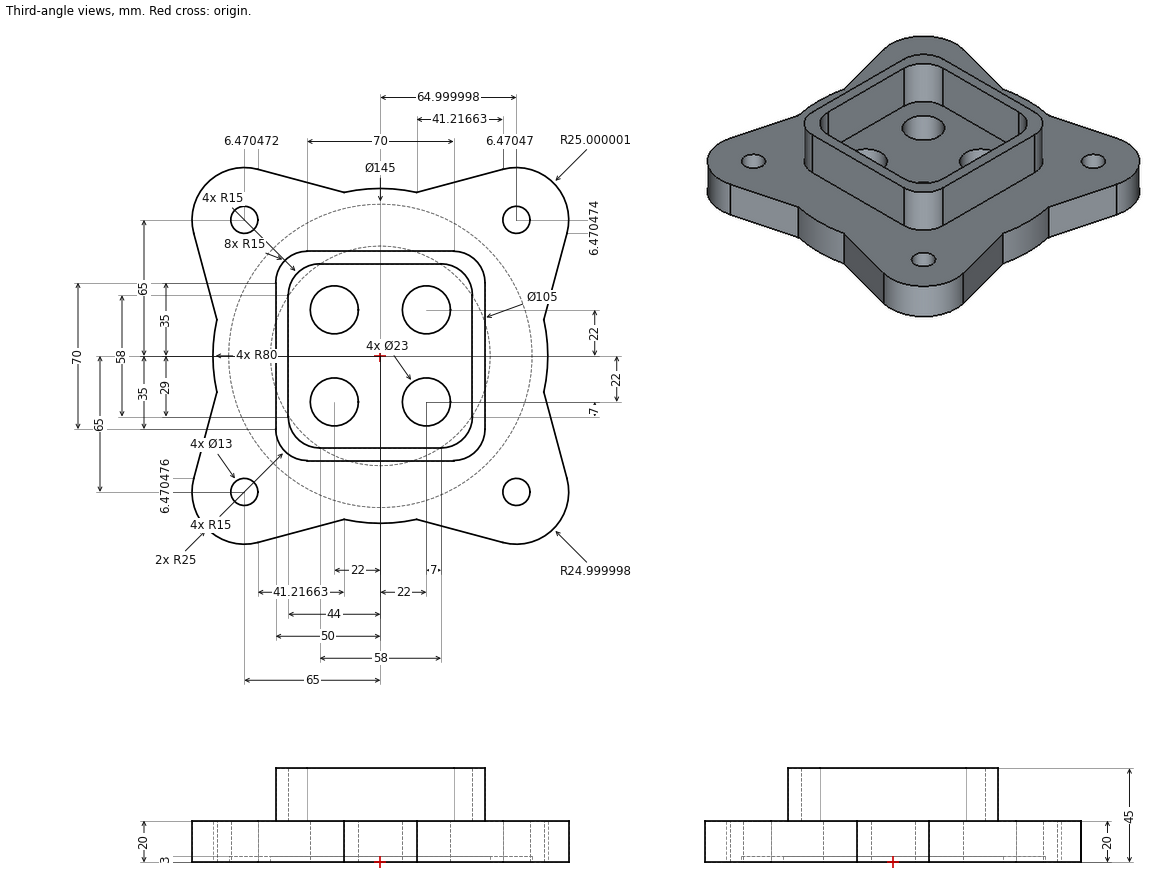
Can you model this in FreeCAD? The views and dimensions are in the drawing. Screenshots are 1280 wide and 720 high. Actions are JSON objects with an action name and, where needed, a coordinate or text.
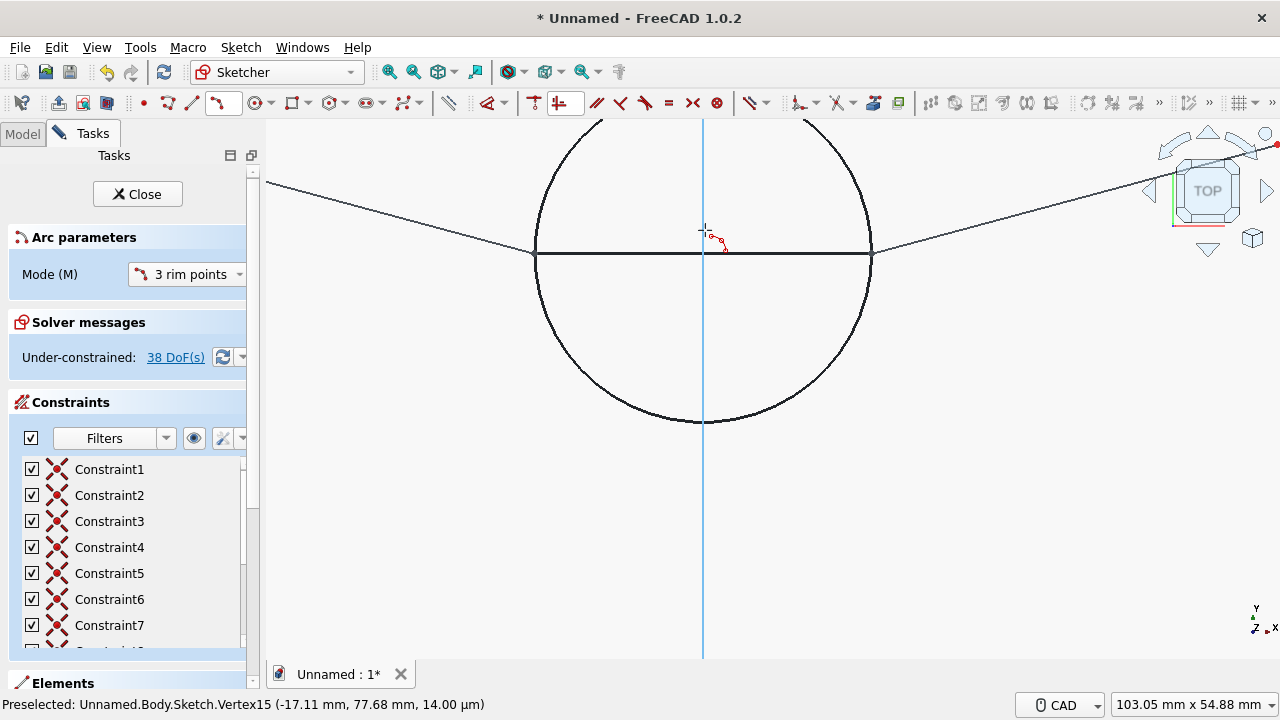
{"action": "left_click", "coordinate": [703, 231]}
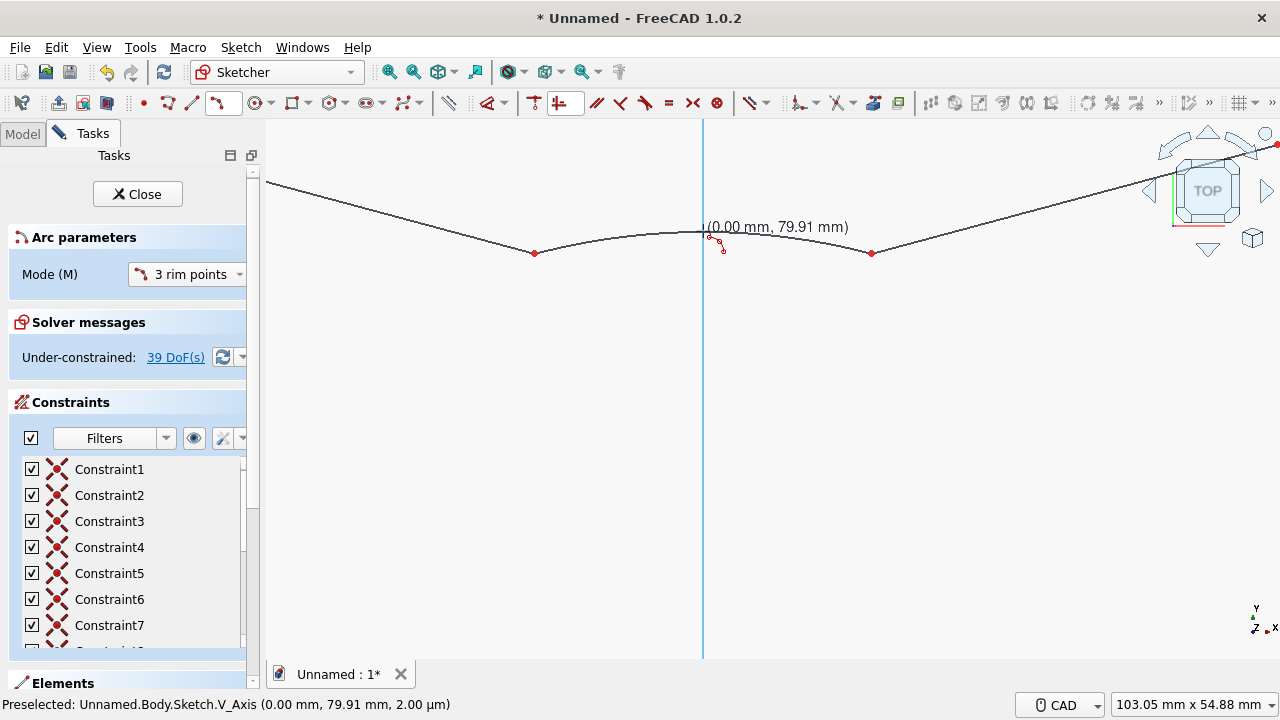
{"action": "scroll", "coordinate": [705, 230], "scroll_direction": "down", "scroll_amount": 8}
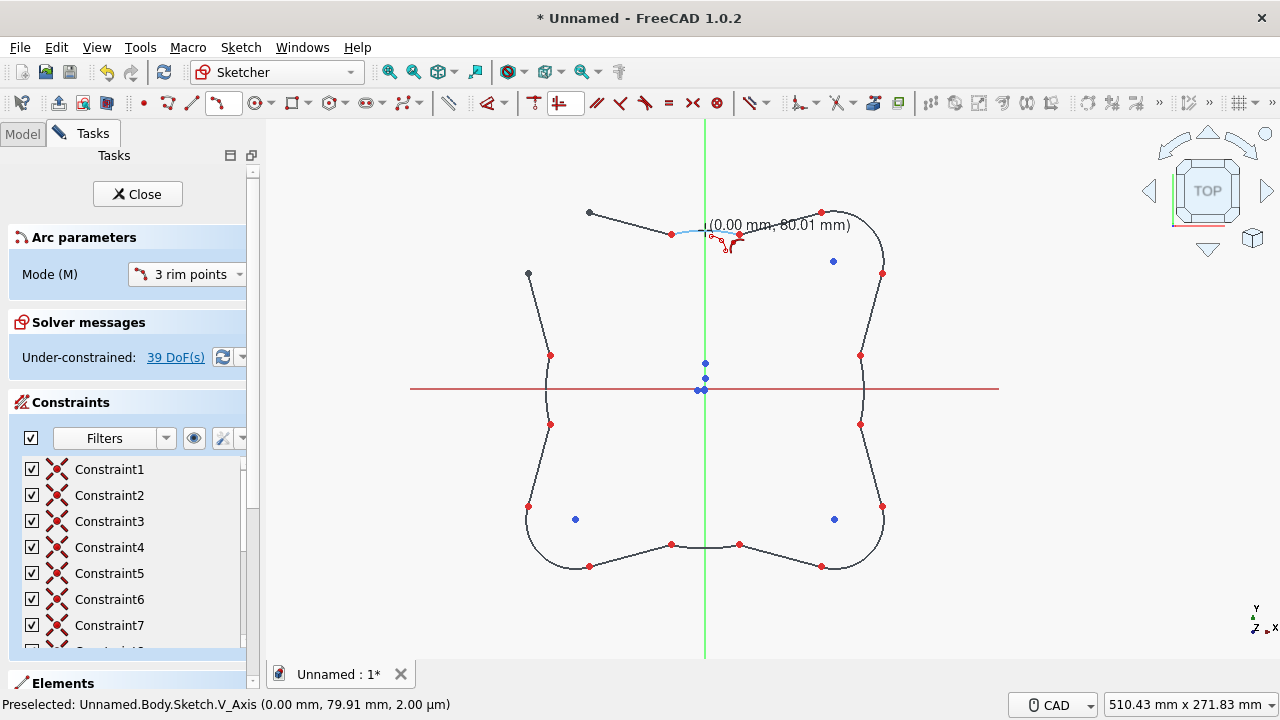
{"action": "left_click", "coordinate": [589, 213]}
{"action": "left_click", "coordinate": [528, 274]}
{"action": "left_click", "coordinate": [541, 225]}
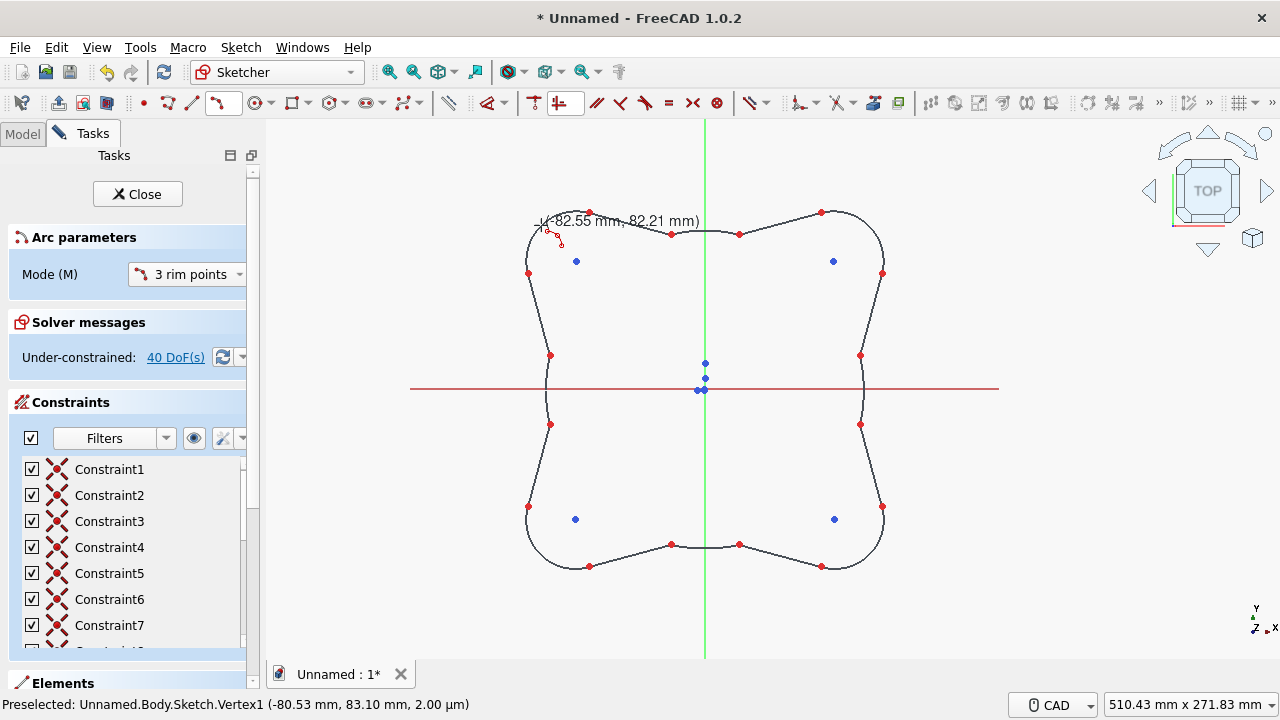
{"action": "left_click", "coordinate": [192, 104]}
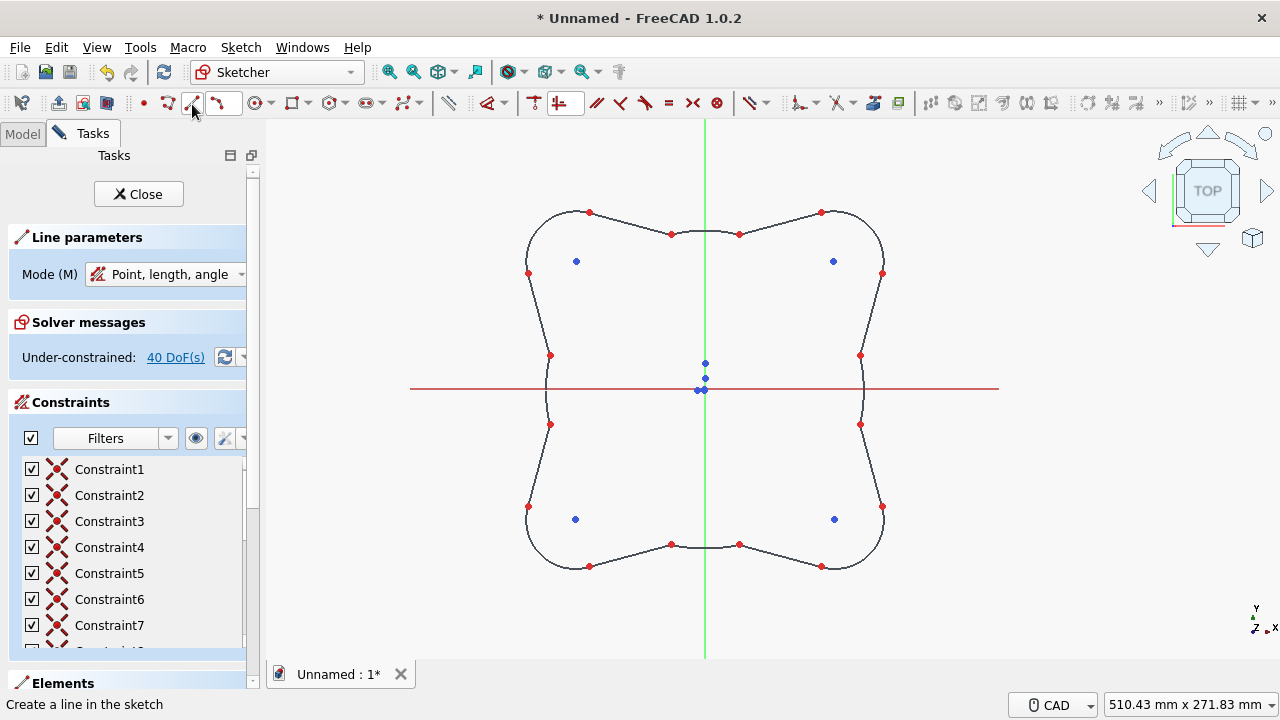
{"action": "left_click", "coordinate": [606, 459]}
{"action": "left_click", "coordinate": [606, 320]}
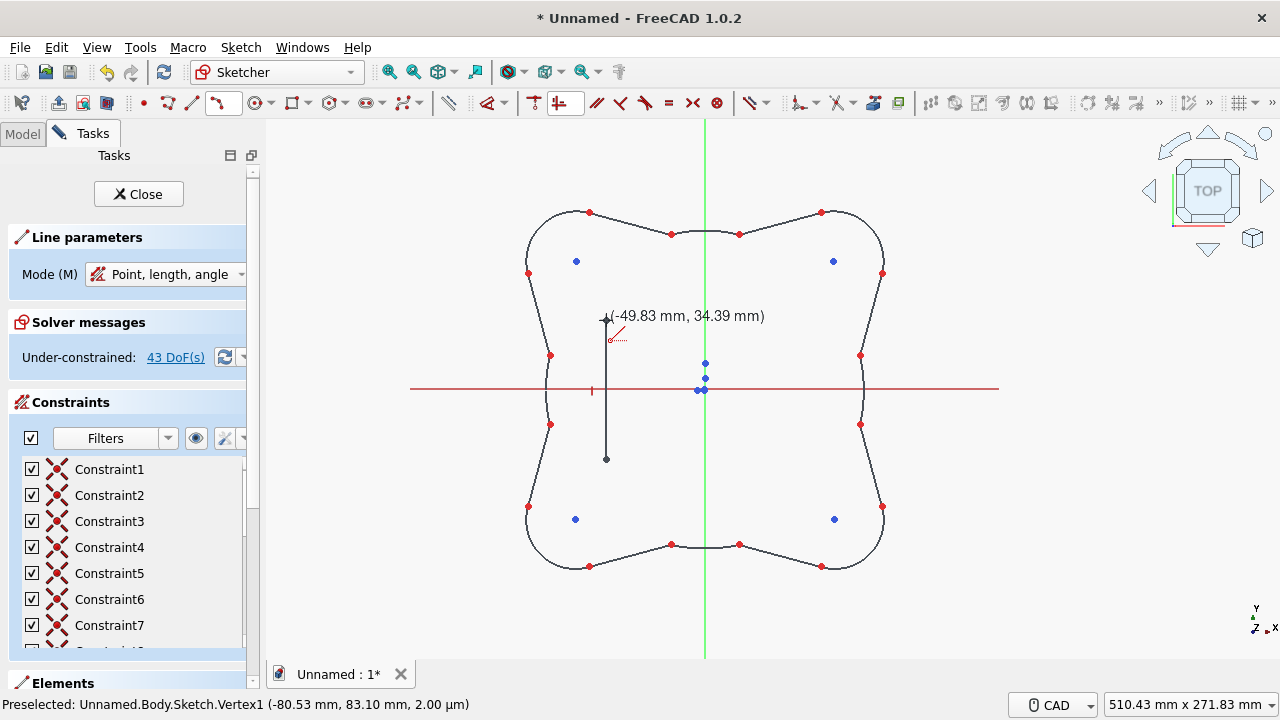
{"action": "left_click", "coordinate": [635, 290]}
{"action": "left_click", "coordinate": [775, 290]}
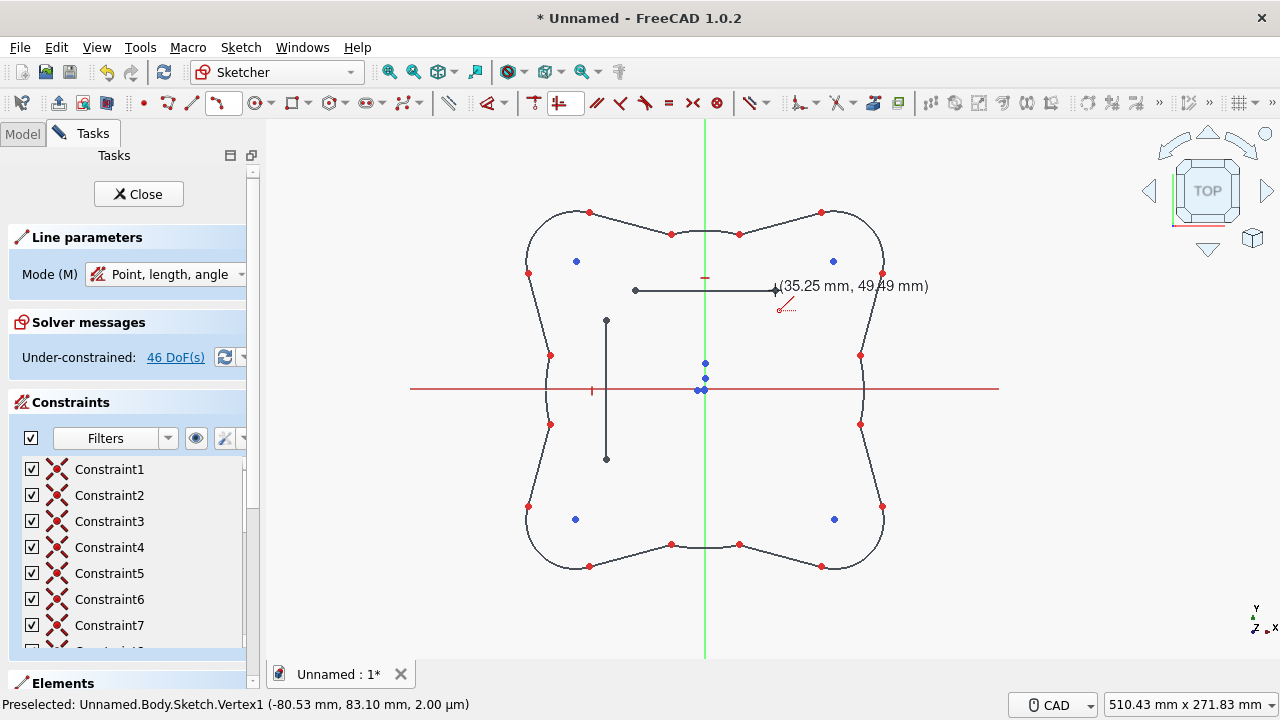
{"action": "left_click", "coordinate": [804, 320]}
{"action": "left_click", "coordinate": [804, 459]}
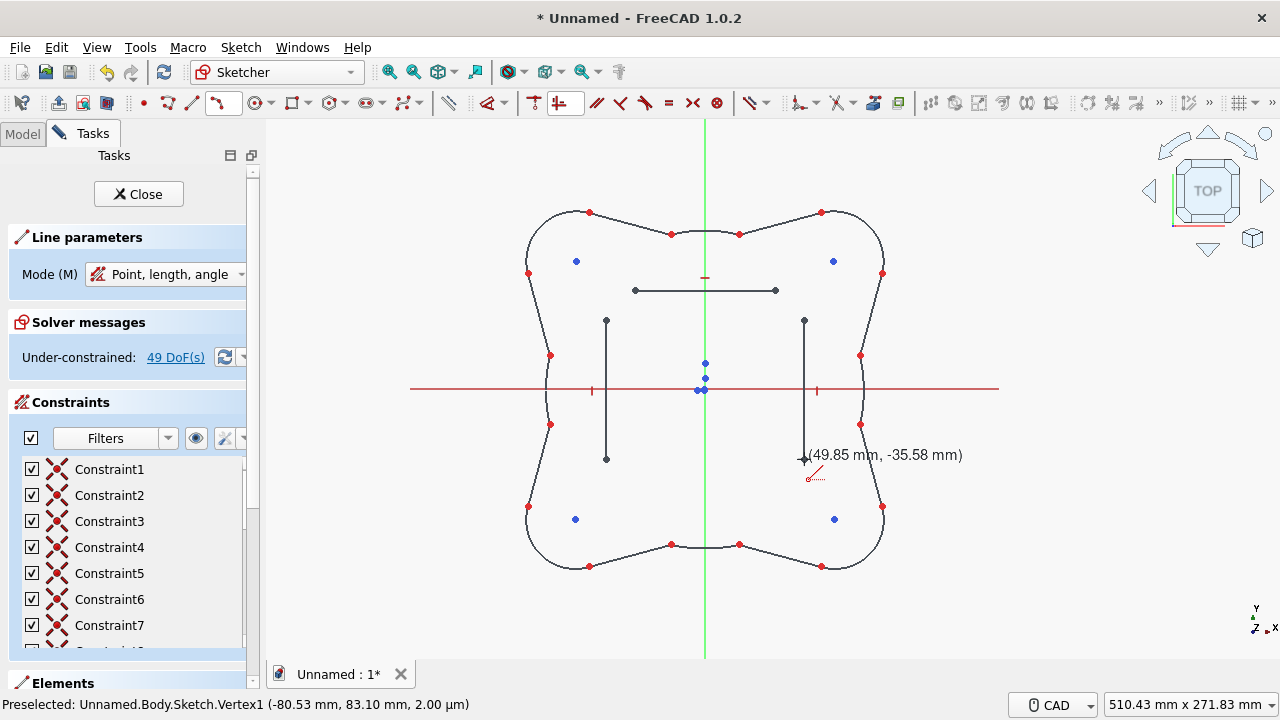
{"action": "left_click", "coordinate": [775, 489]}
{"action": "left_click", "coordinate": [635, 489]}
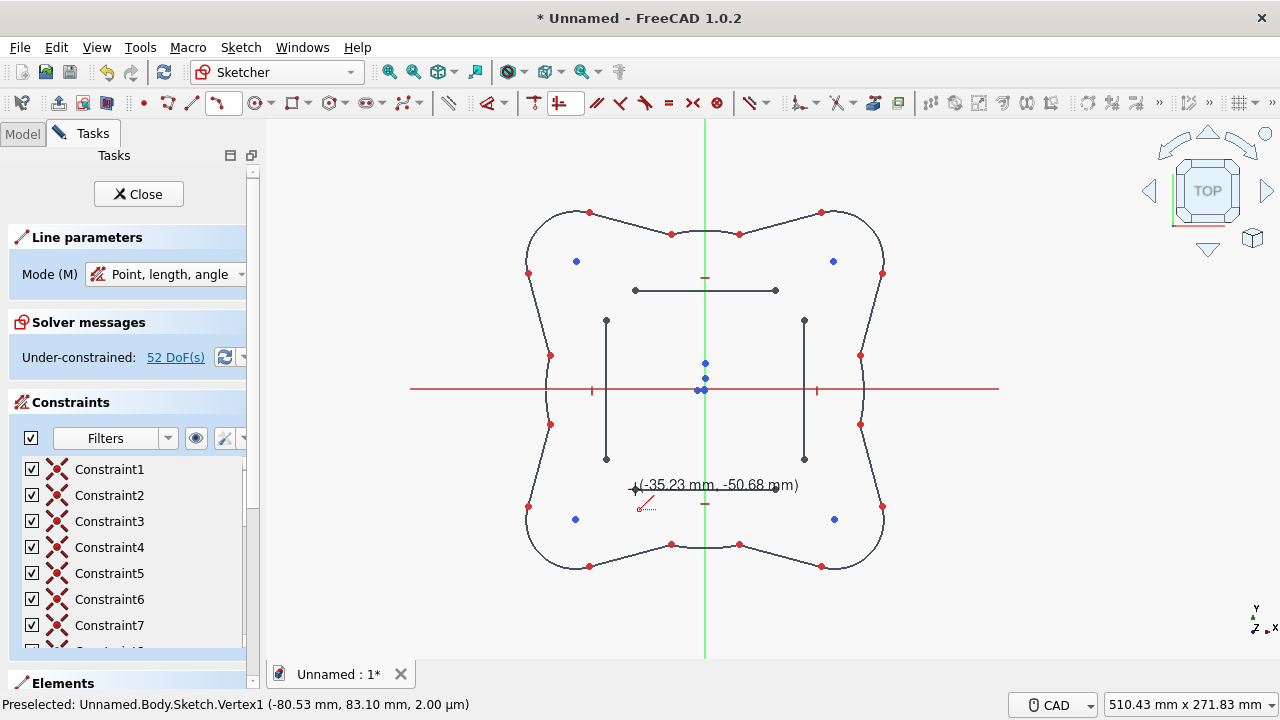
{"action": "key", "text": "g 3 a"}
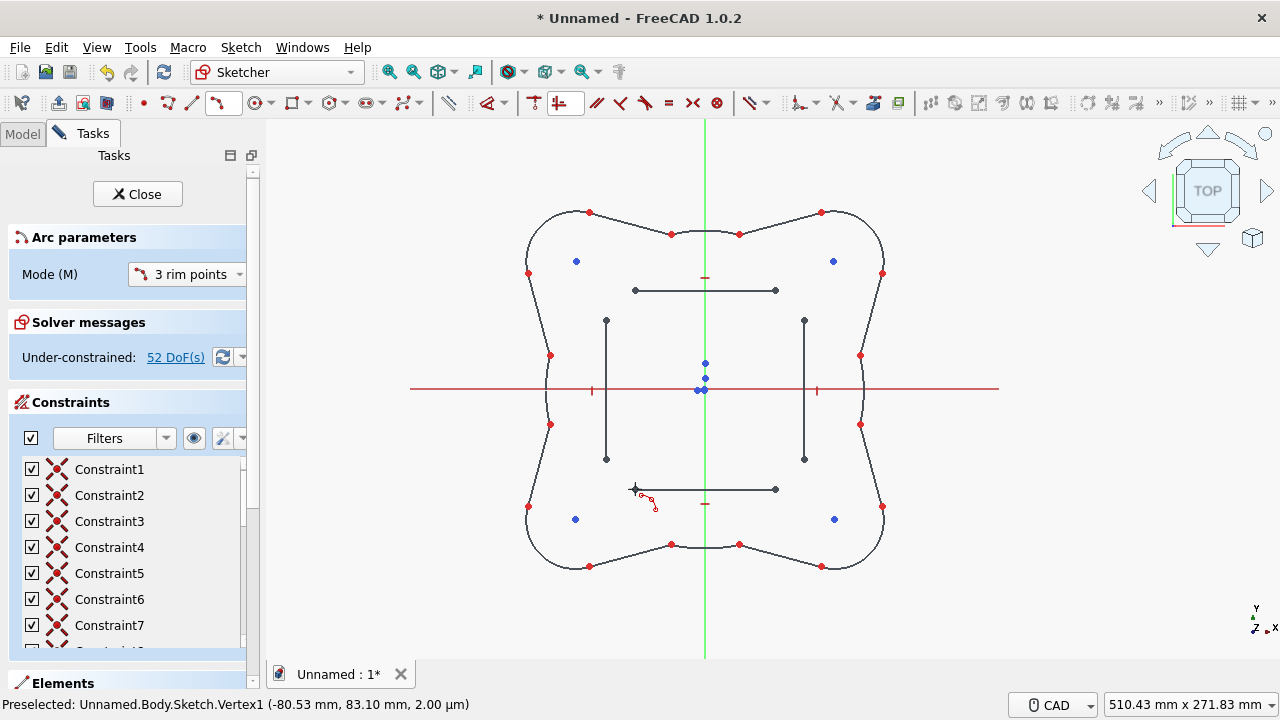
{"action": "left_click", "coordinate": [606, 321]}
{"action": "left_click", "coordinate": [635, 291]}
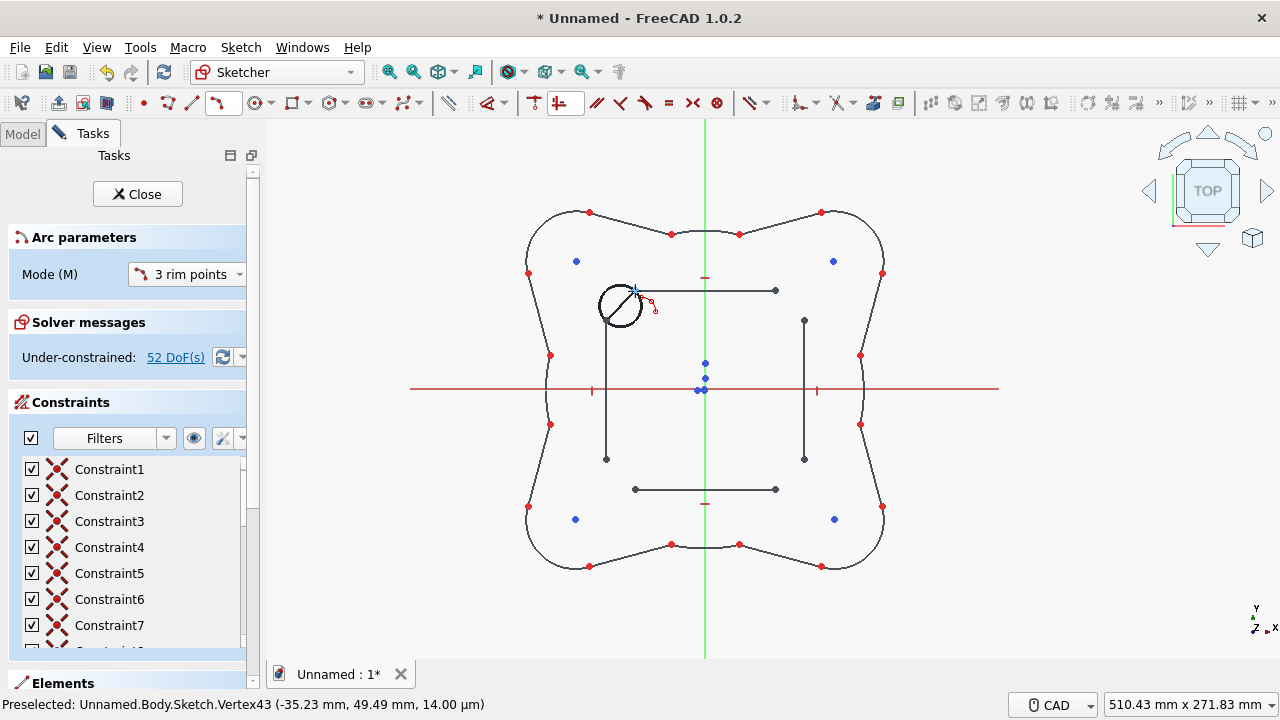
{"action": "scroll", "coordinate": [614, 299], "scroll_direction": "up", "scroll_amount": 3}